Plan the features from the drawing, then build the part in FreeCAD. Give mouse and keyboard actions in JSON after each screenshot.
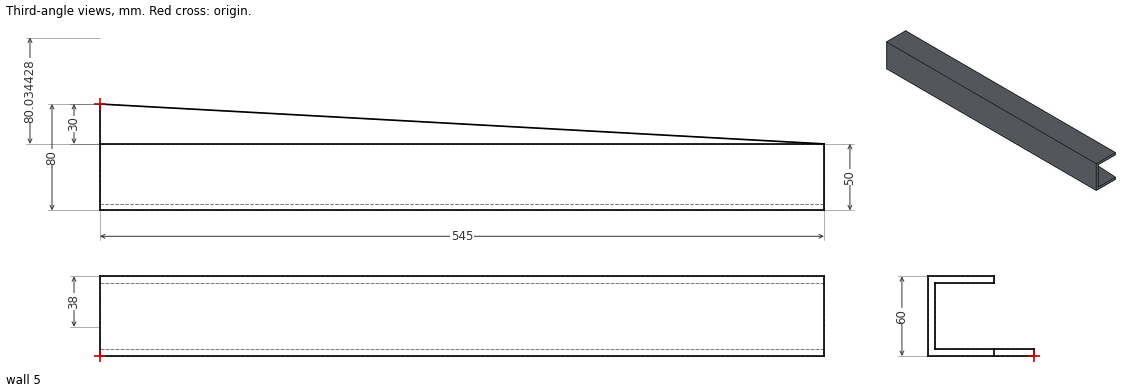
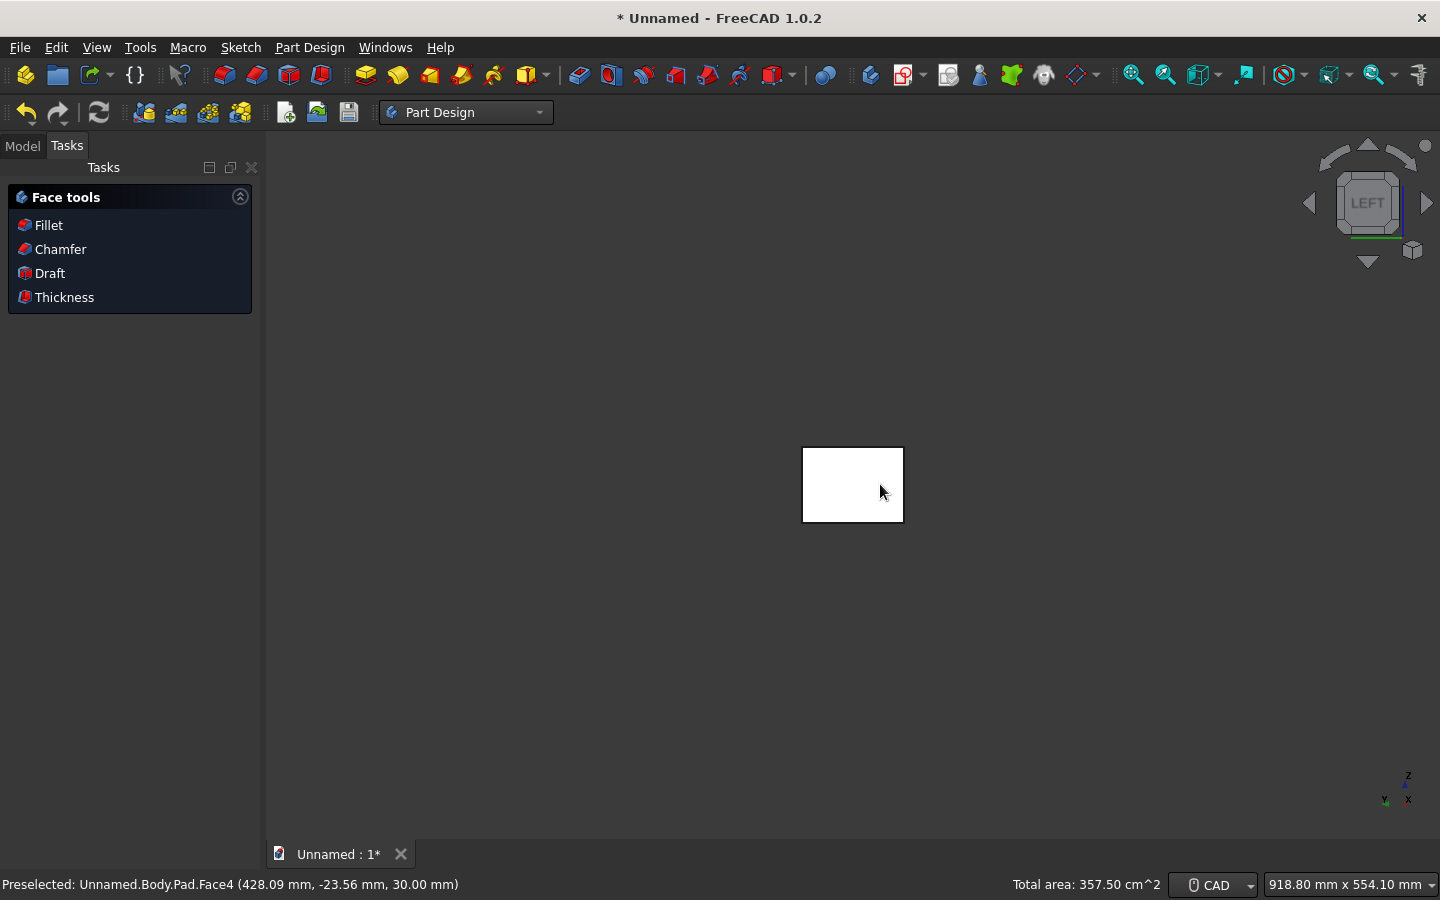
{"action": "left_click", "coordinate": [853, 484], "text": "ctrl"}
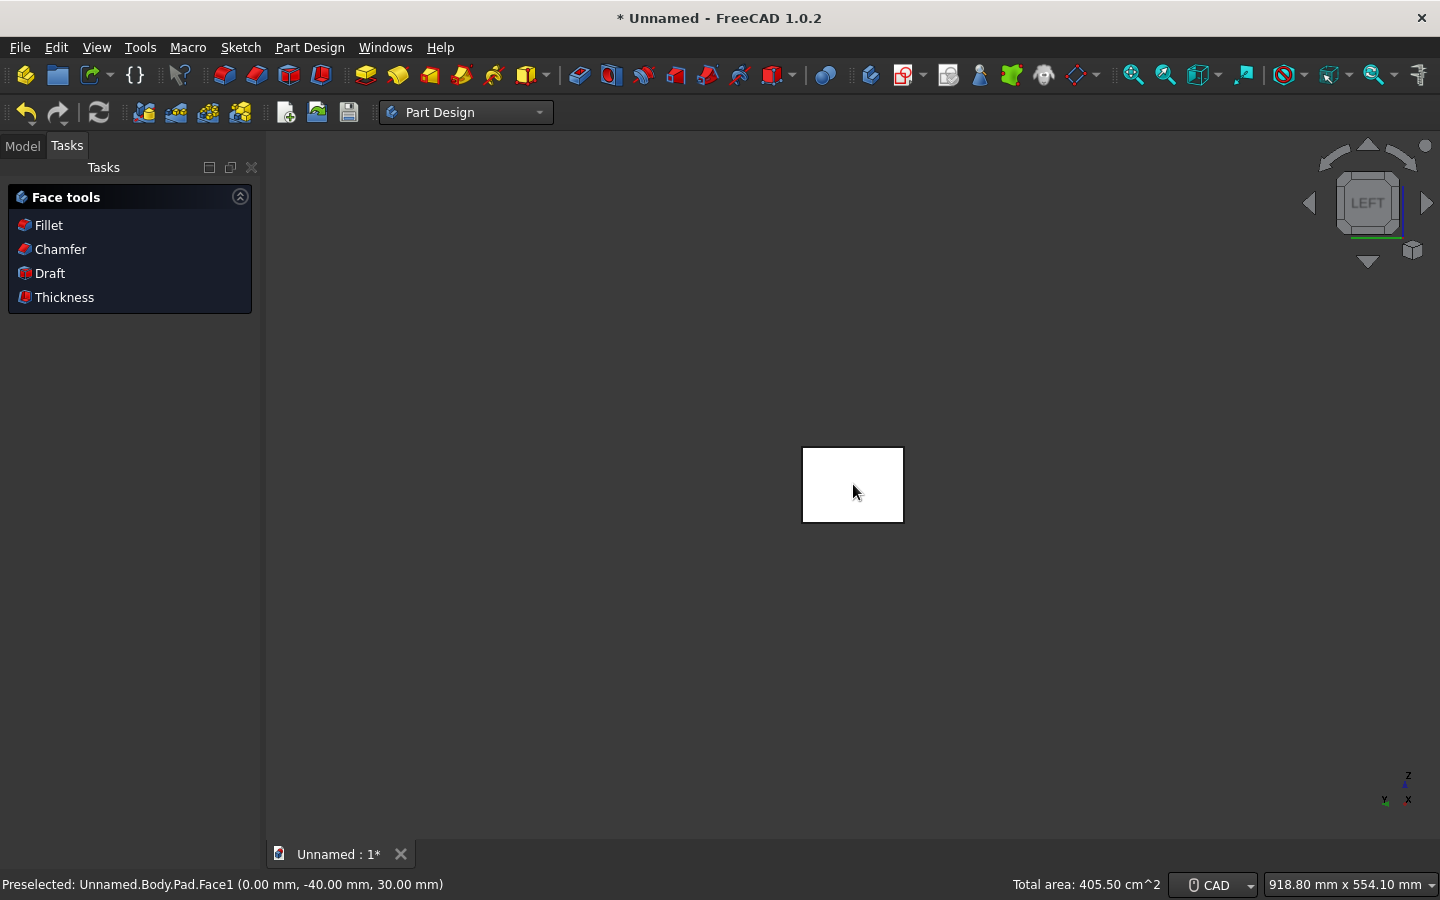
{"action": "left_click", "coordinate": [322, 76]}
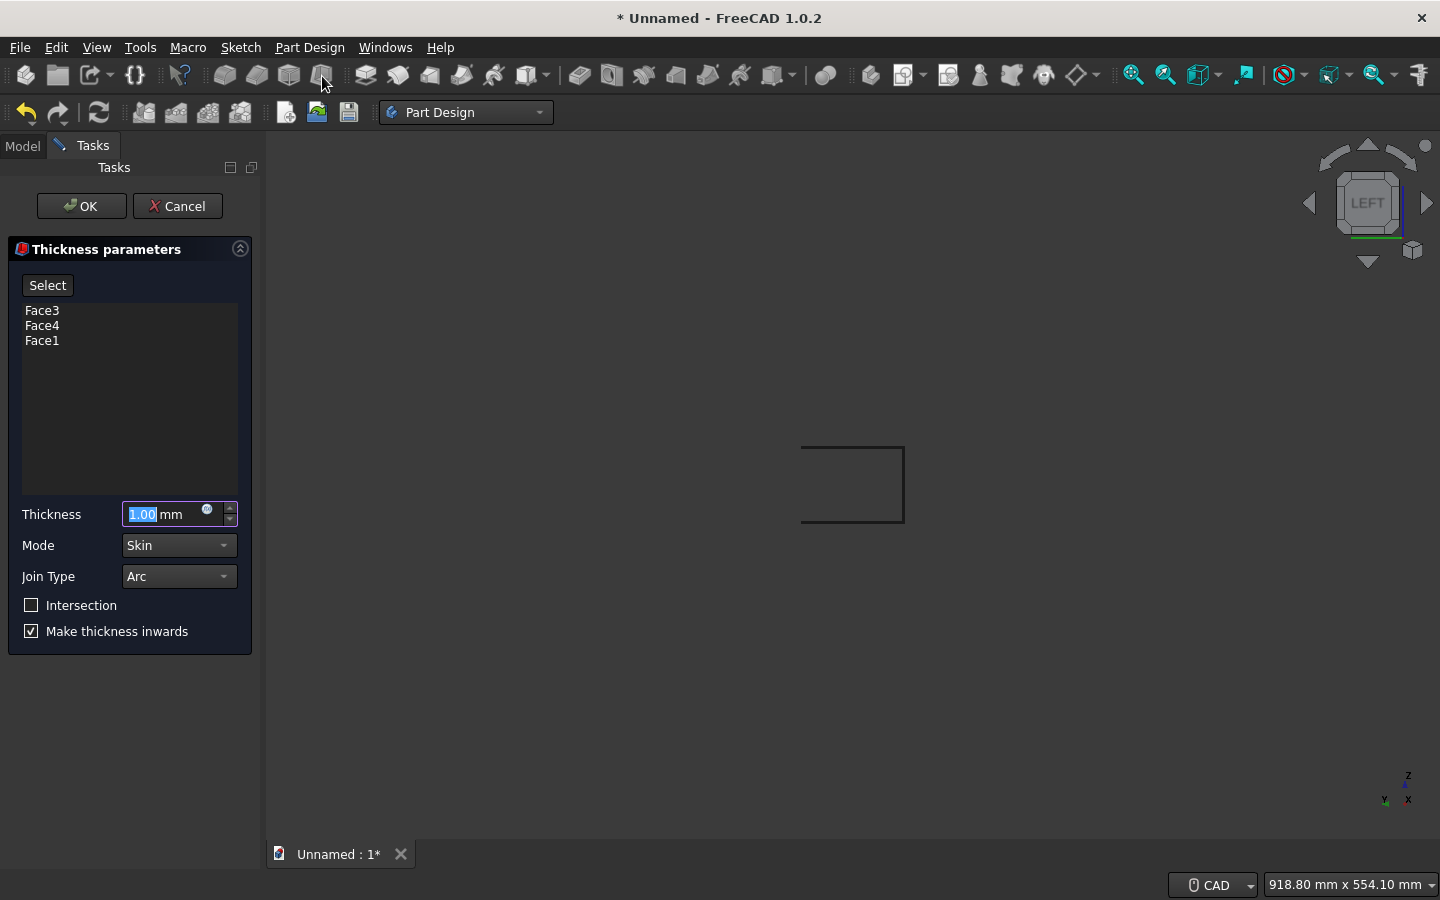
{"action": "type", "text": "5"}
{"action": "key", "text": "Tab"}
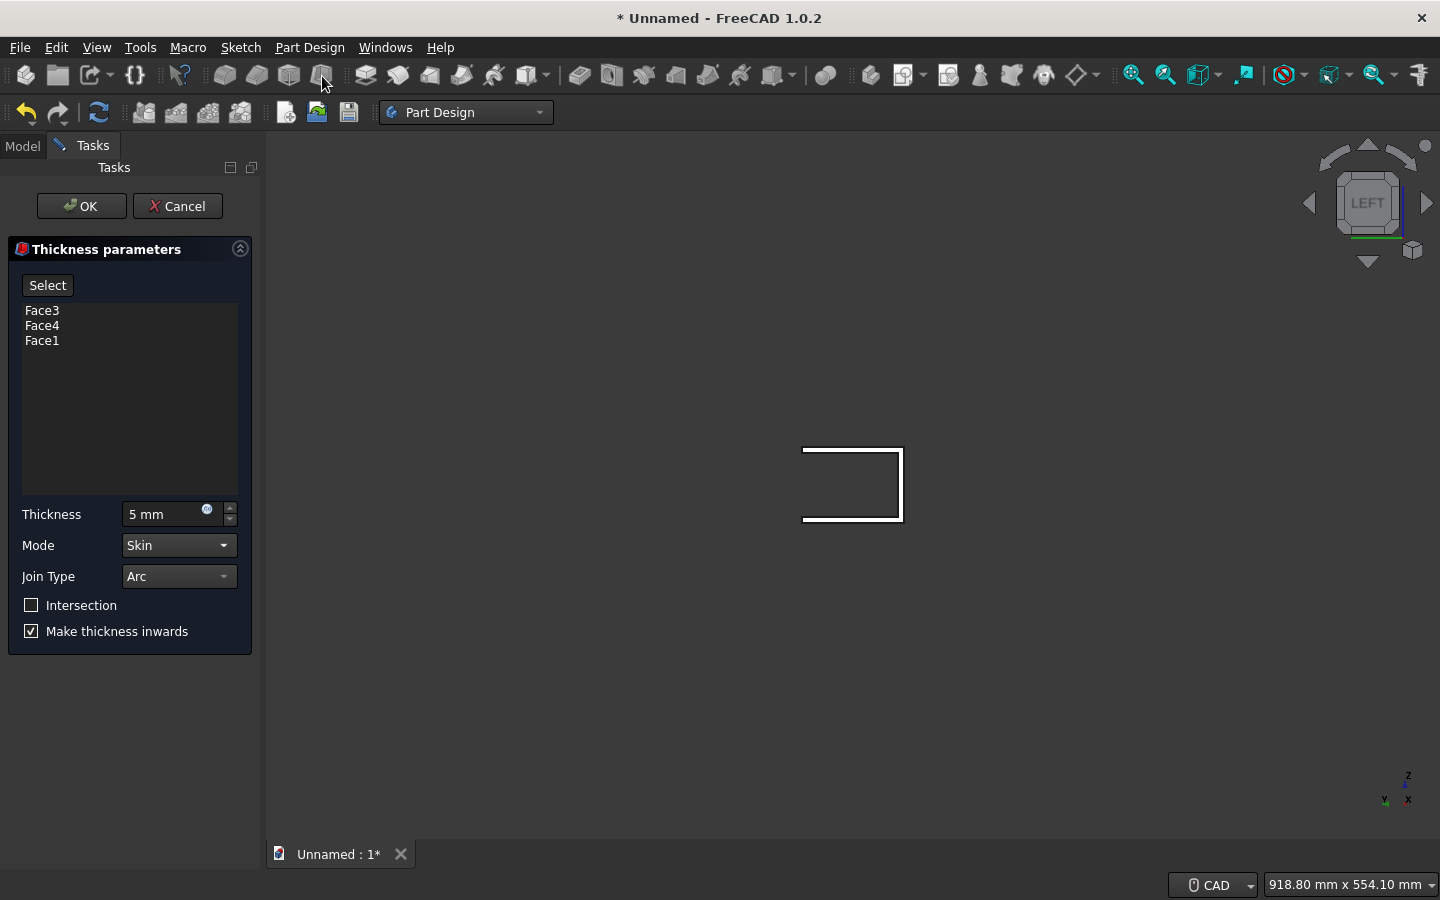
{"action": "left_click", "coordinate": [180, 576]}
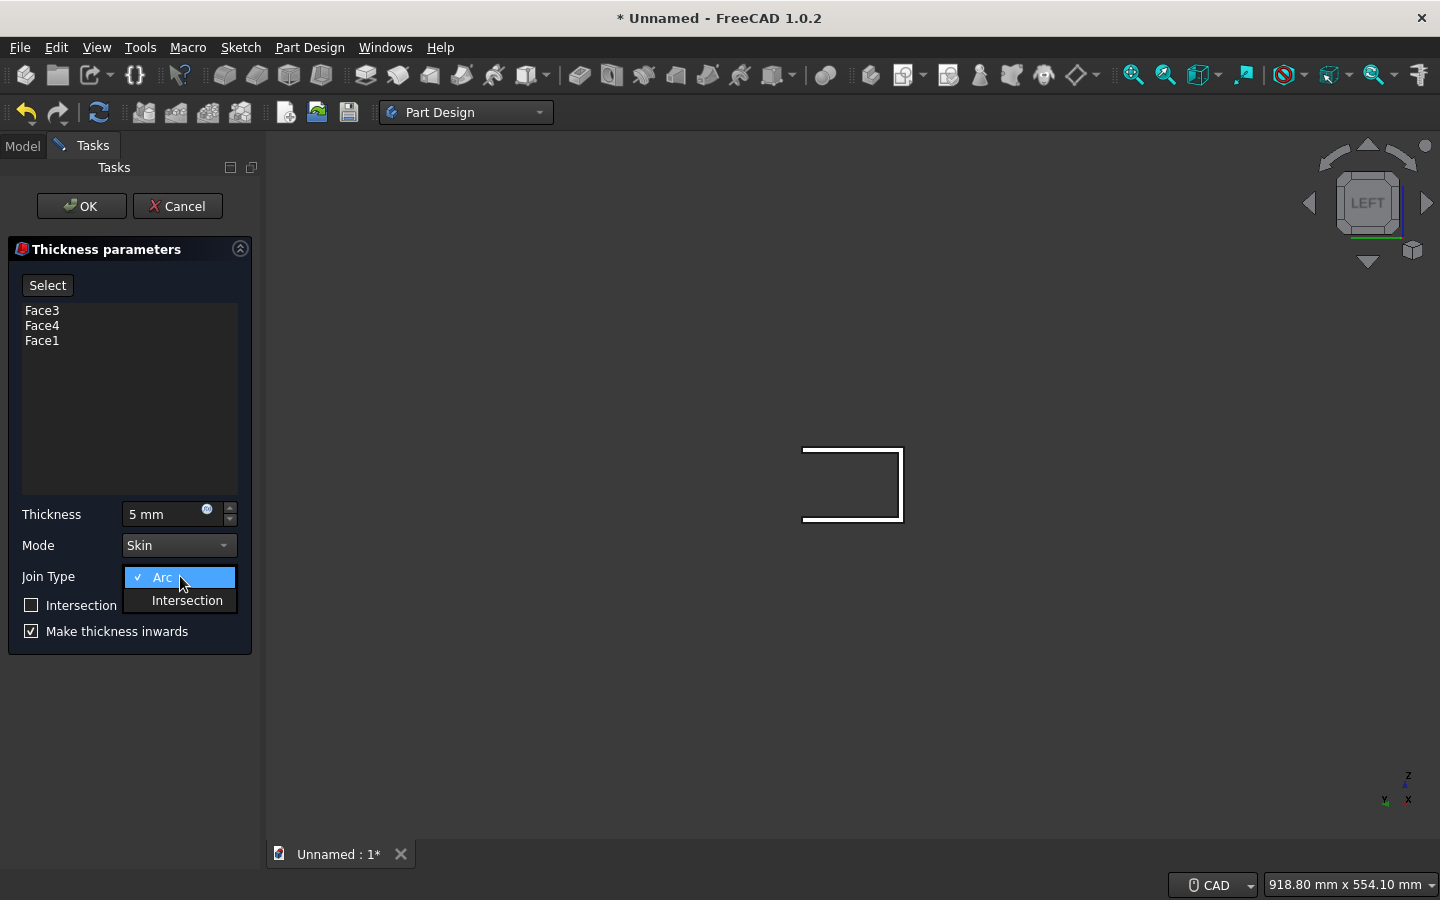
{"action": "left_click", "coordinate": [179, 600]}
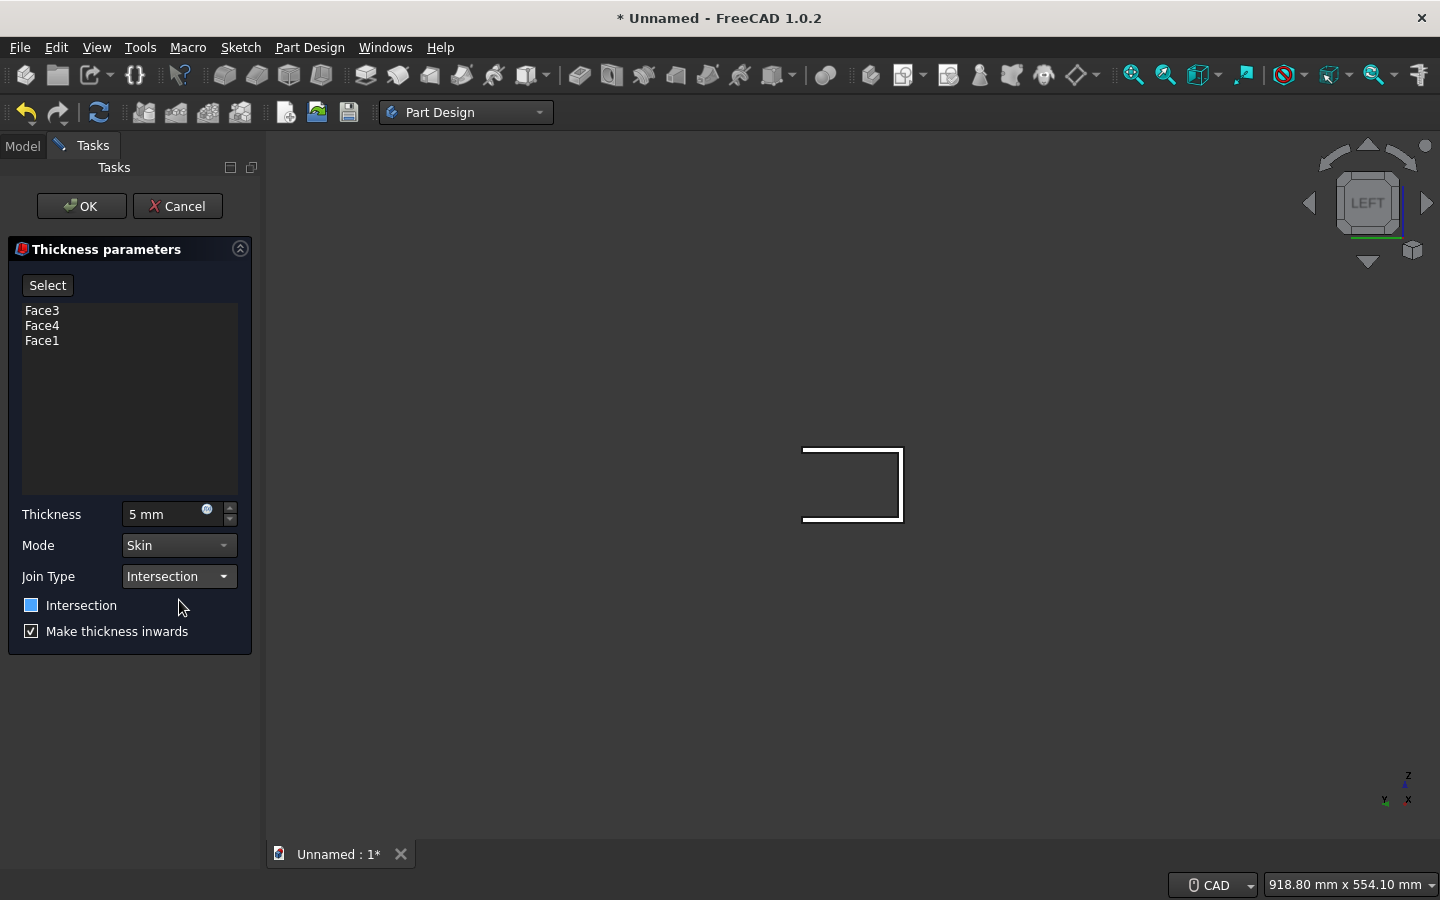
{"action": "left_click", "coordinate": [82, 206]}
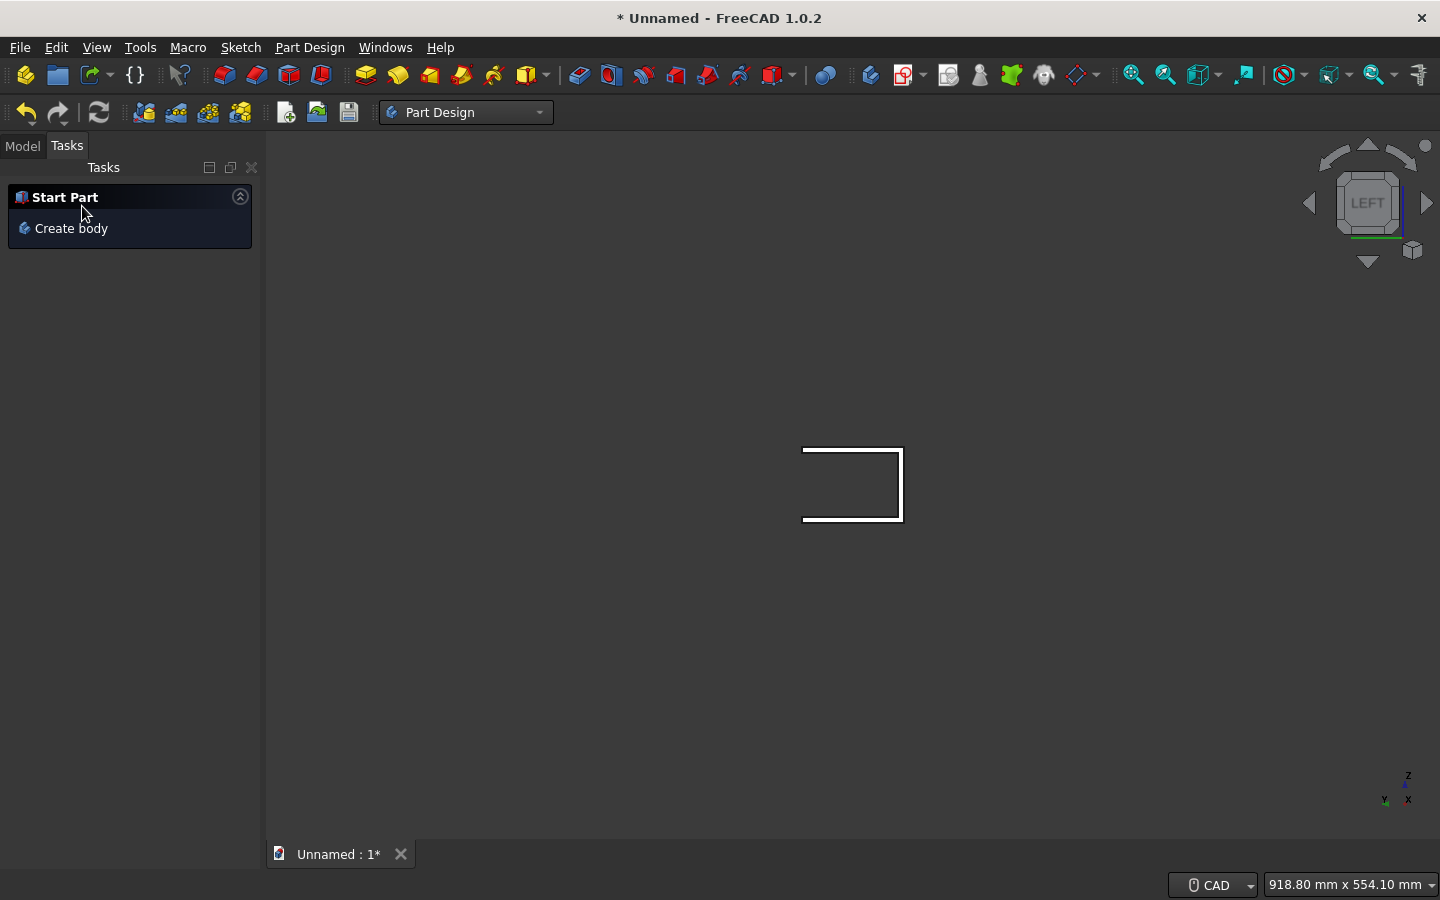
{"action": "left_click", "coordinate": [1134, 76]}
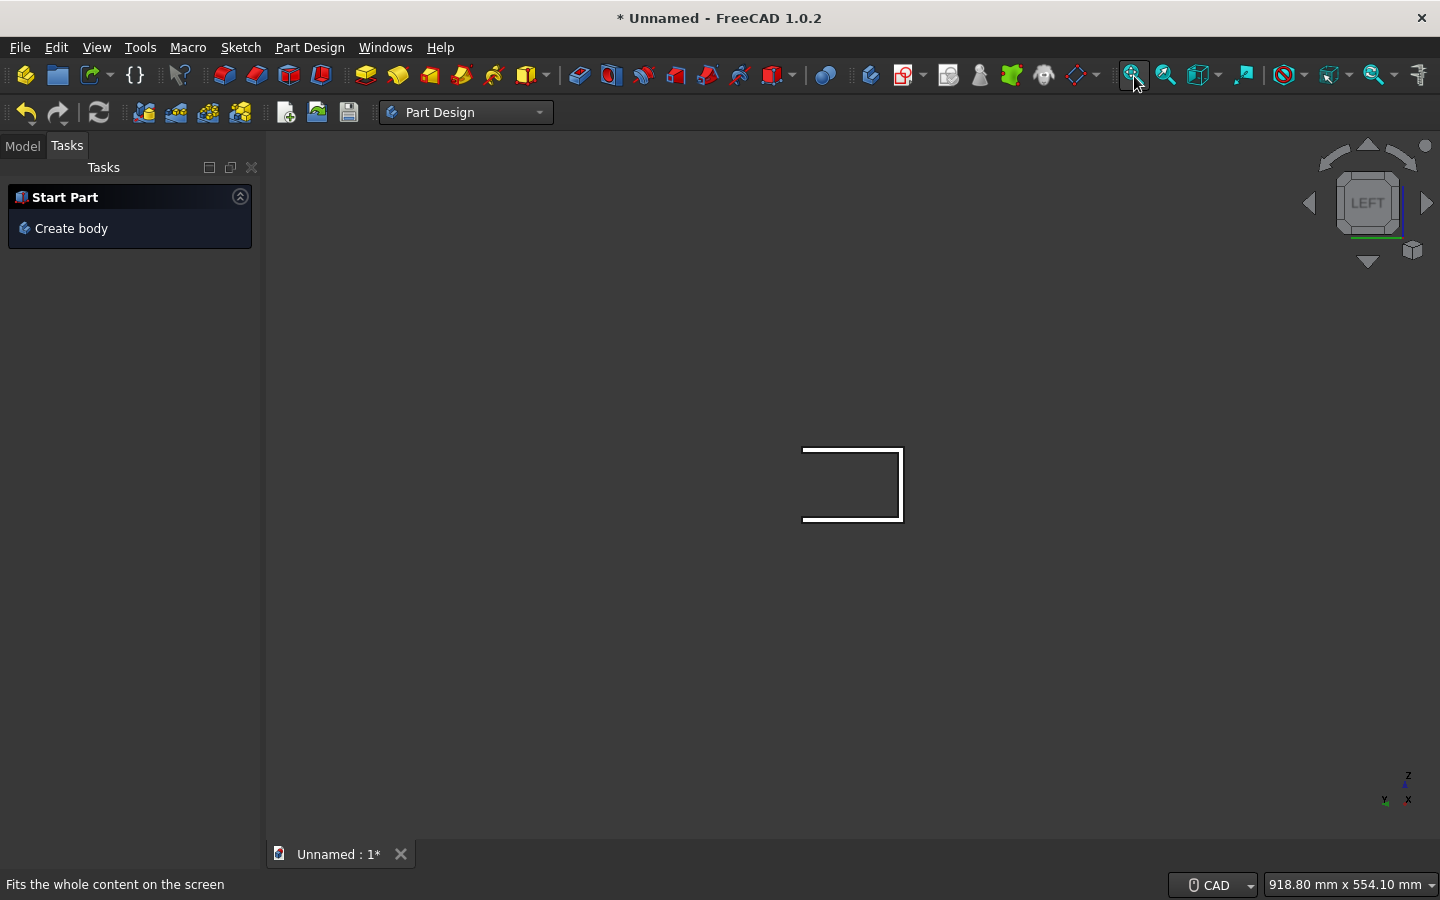
{"action": "key", "text": "0"}